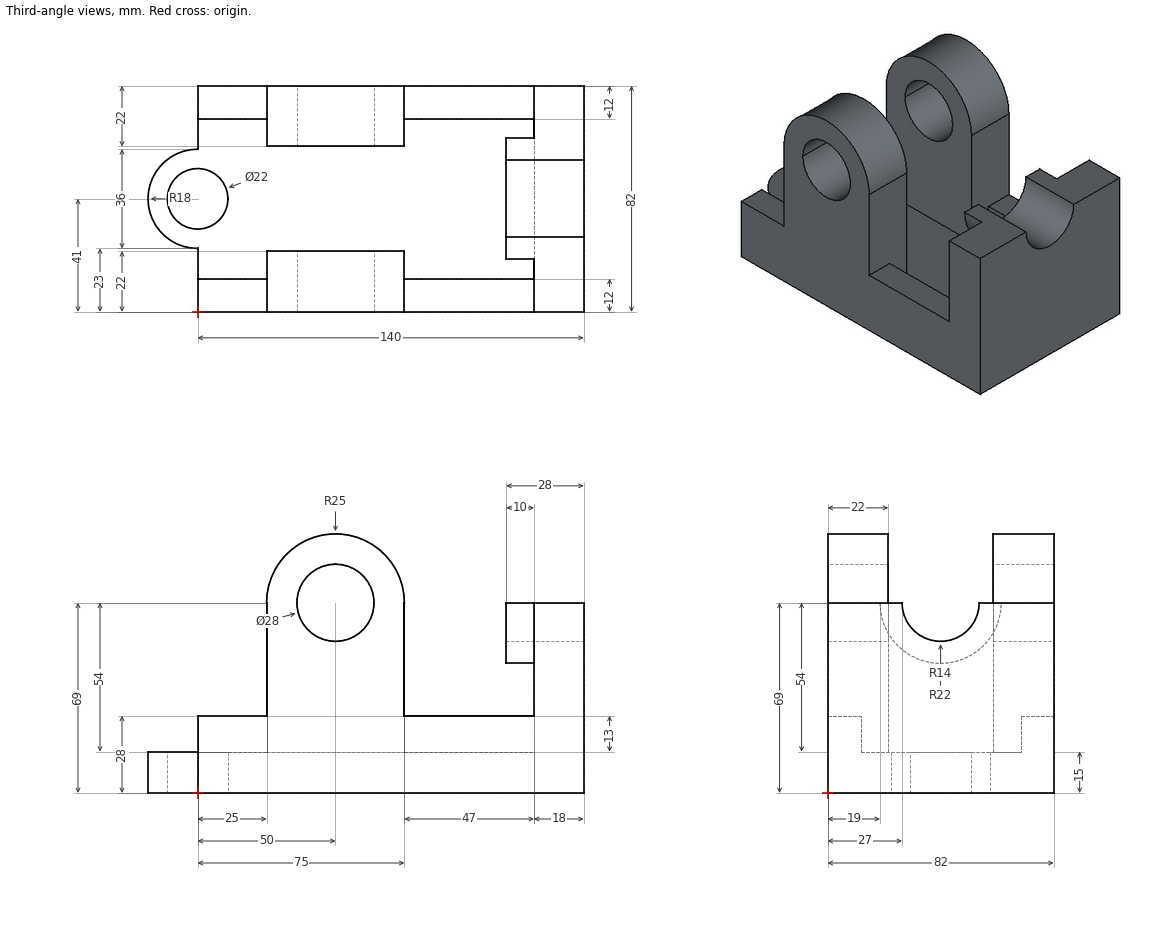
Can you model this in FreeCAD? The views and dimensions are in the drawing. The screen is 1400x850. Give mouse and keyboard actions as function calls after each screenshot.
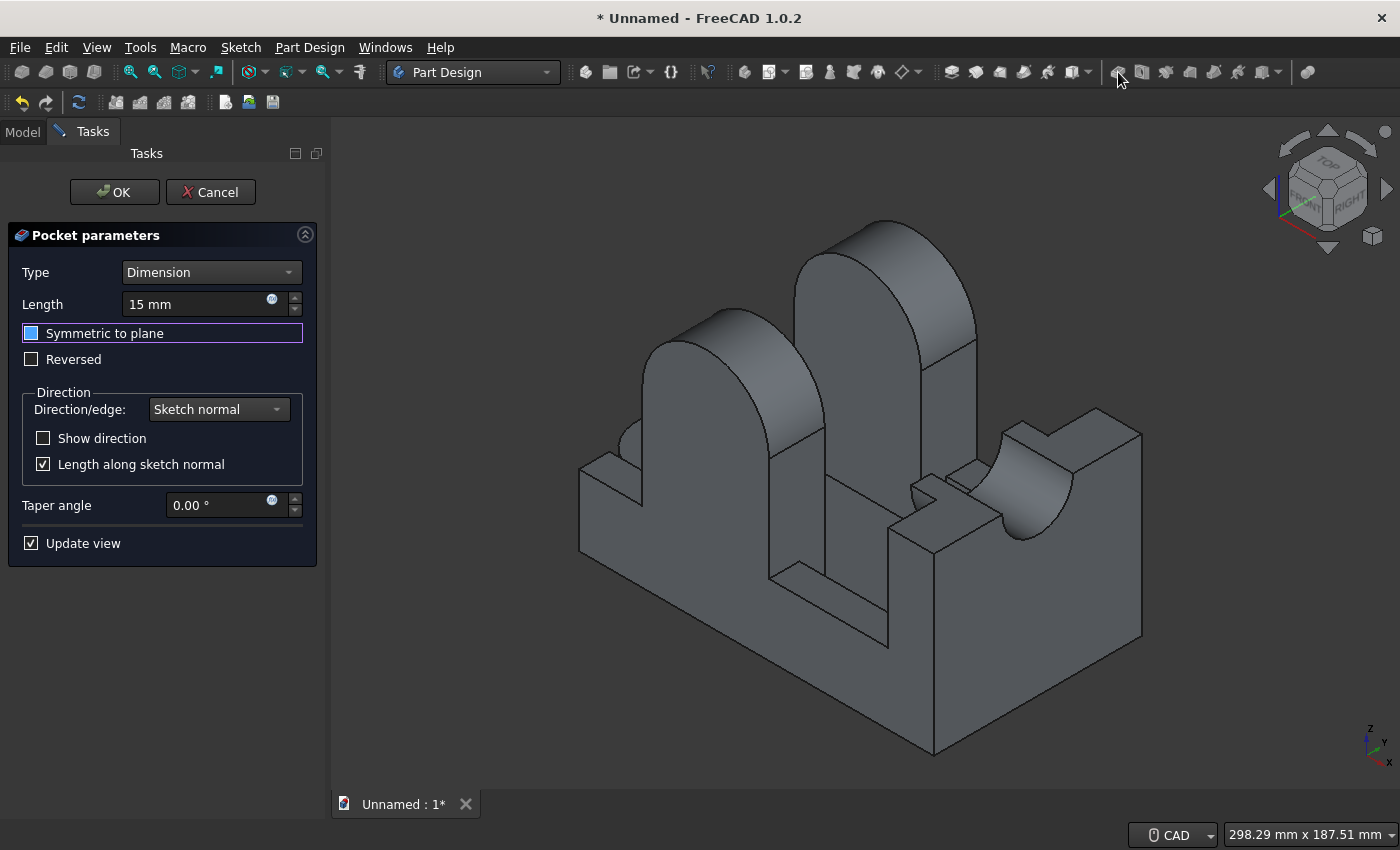
click(115, 192)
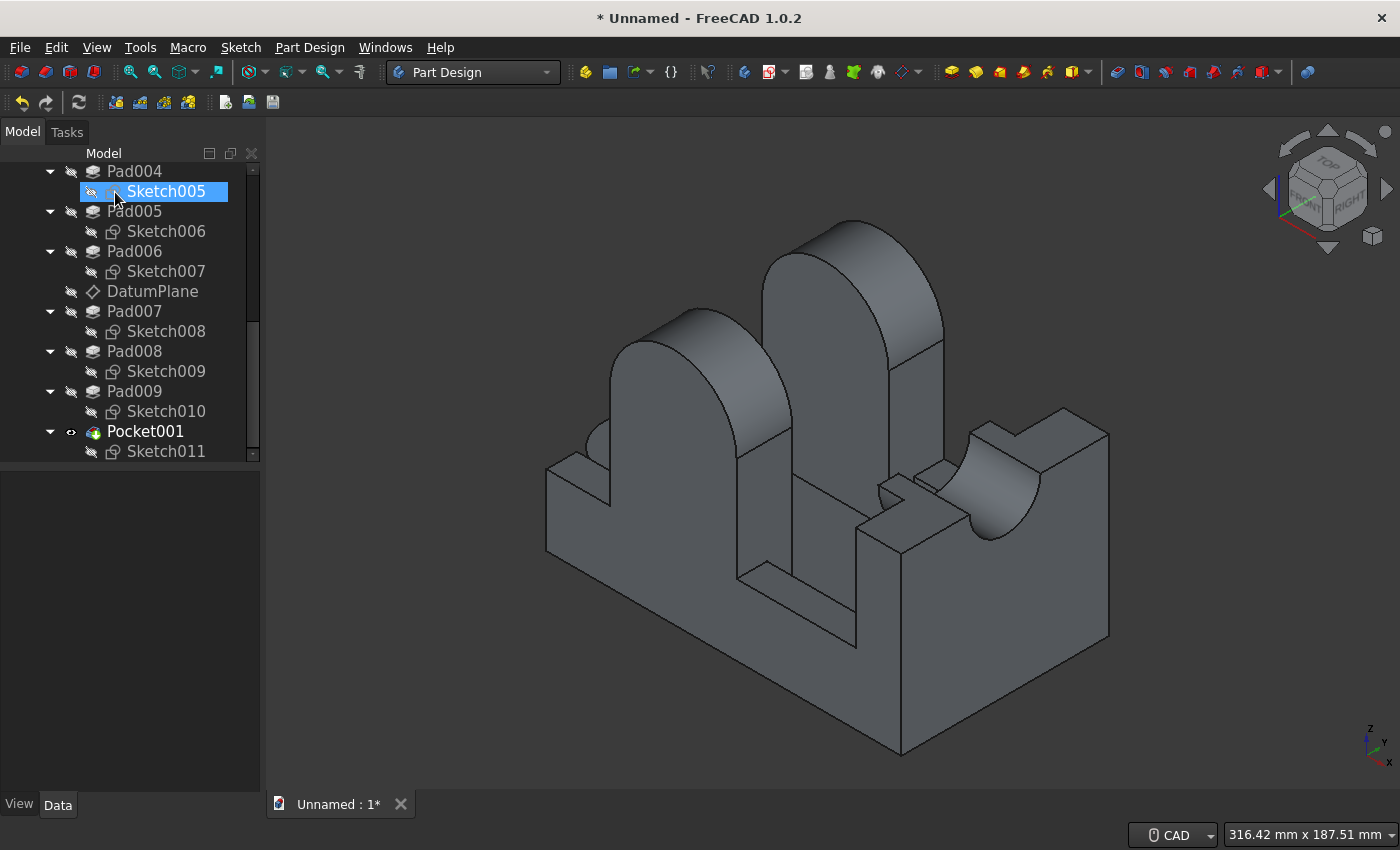
key(4)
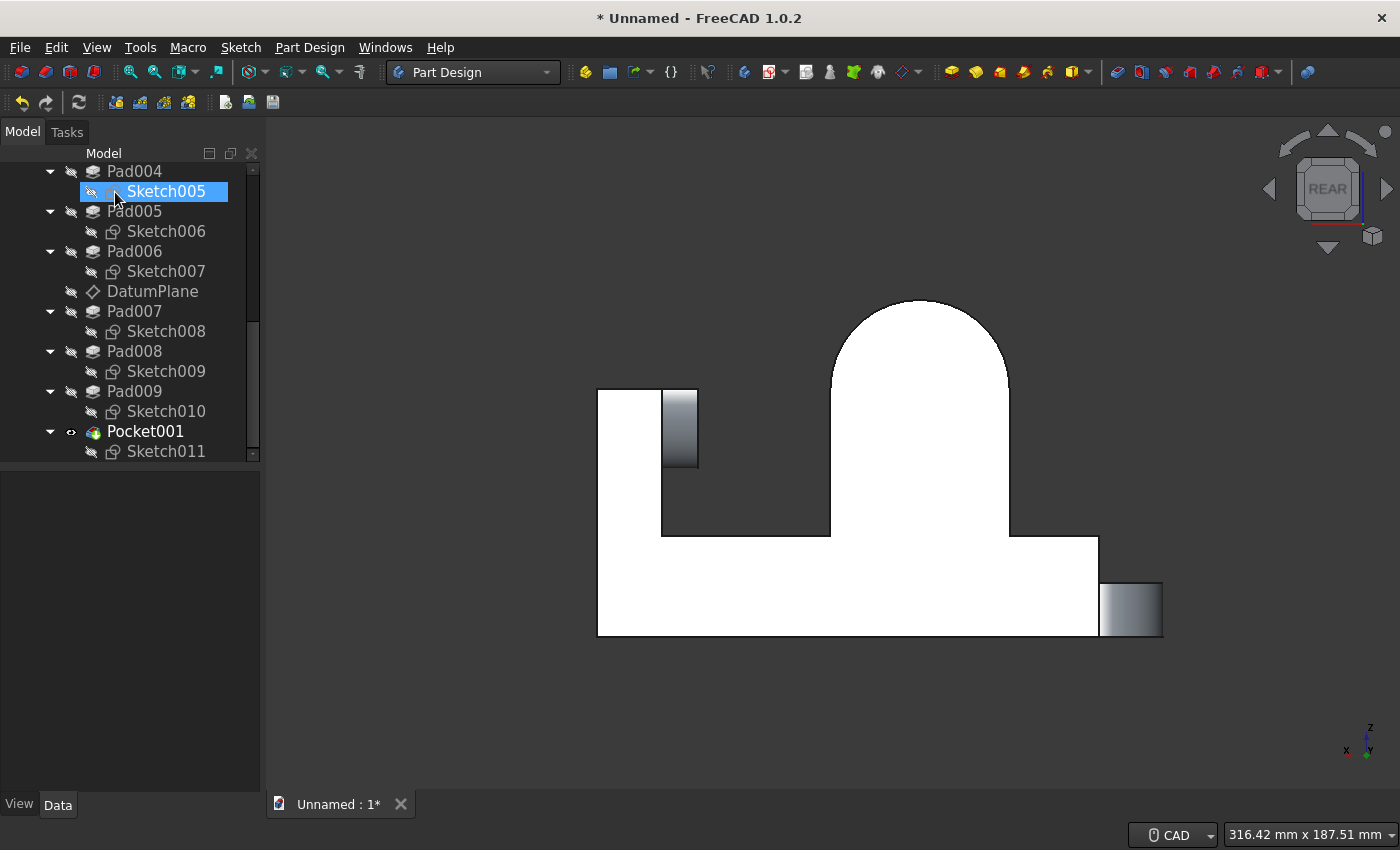
click(920, 419)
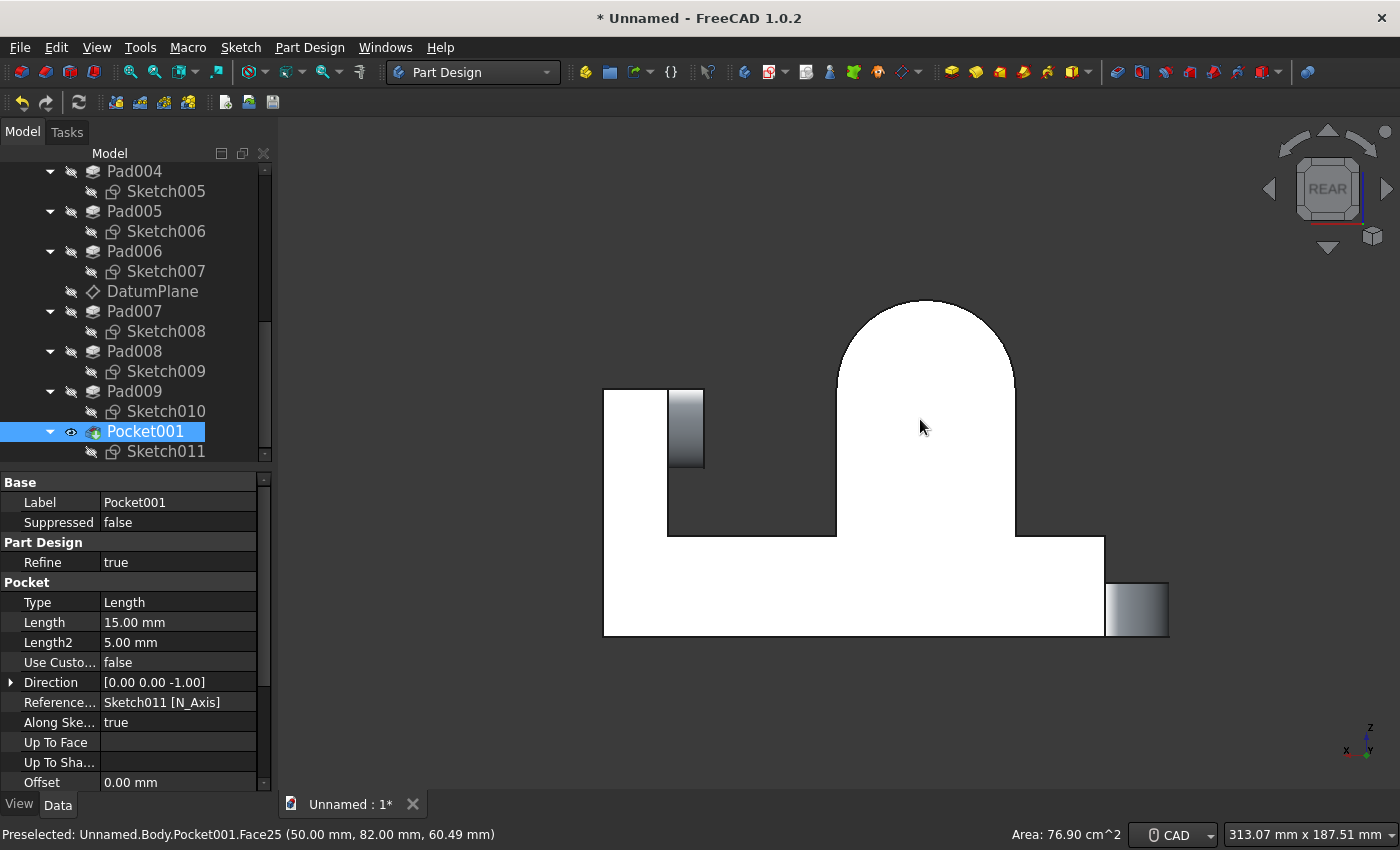
click(770, 72)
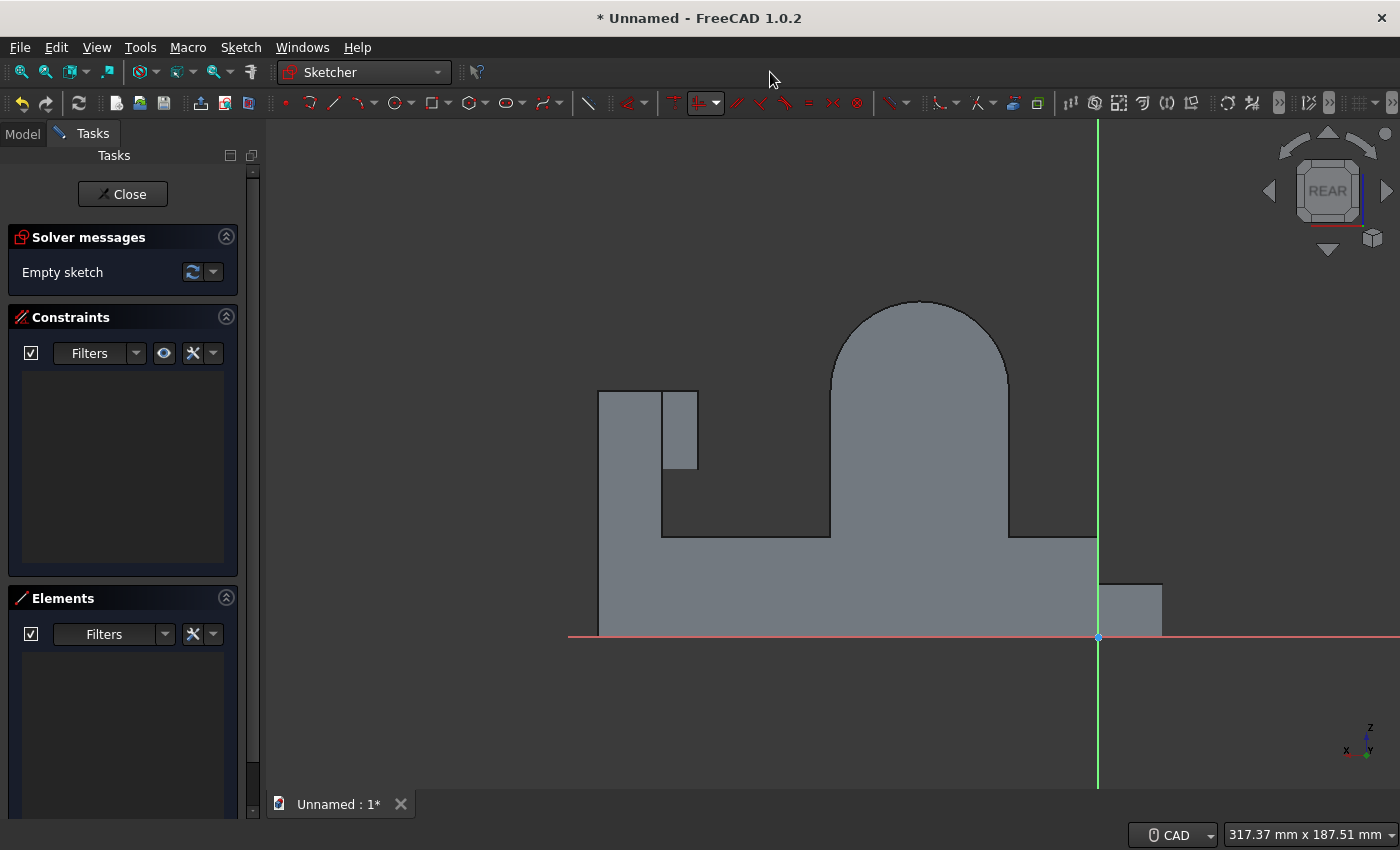
scroll(971, 370, up, 7)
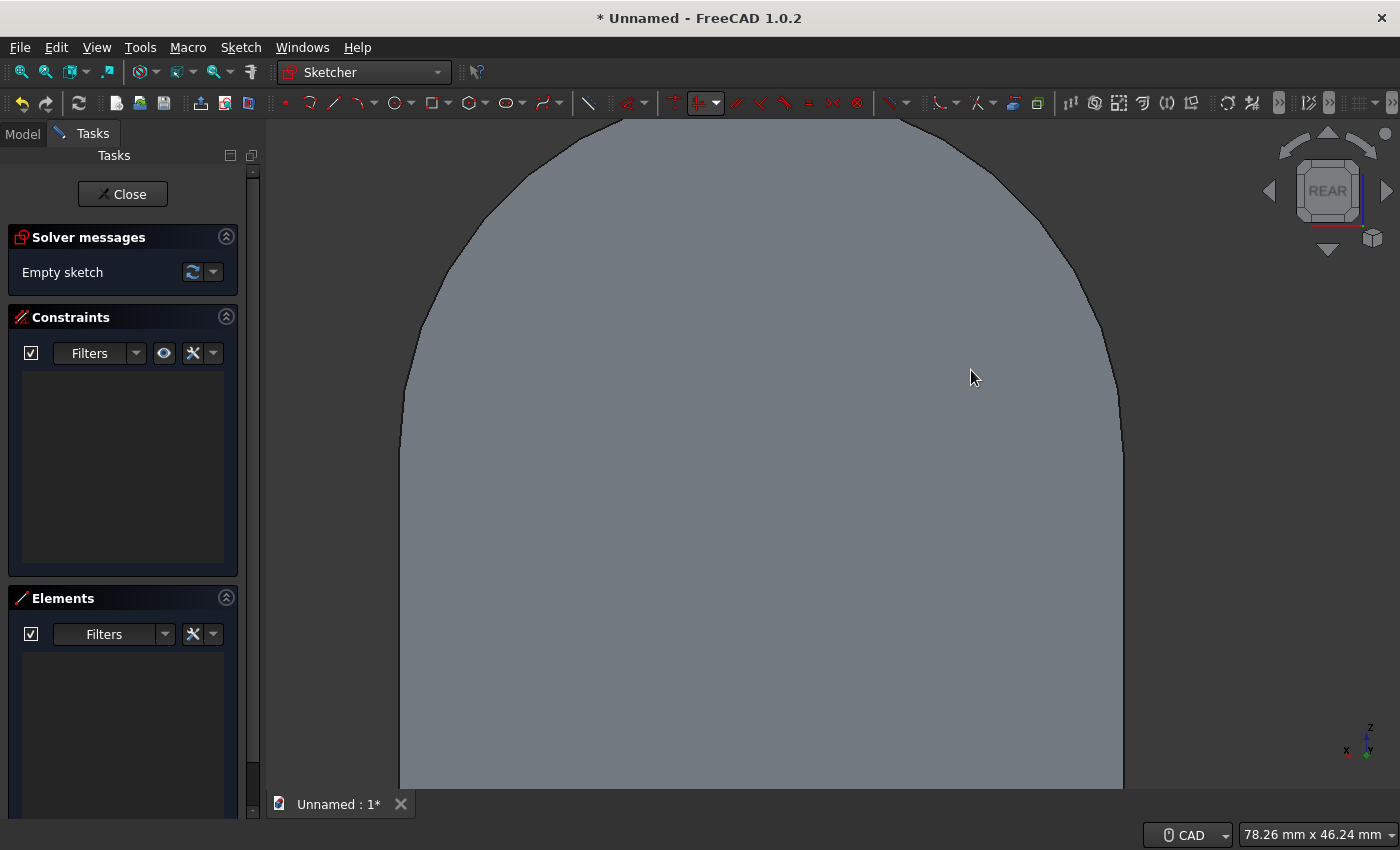
click(396, 104)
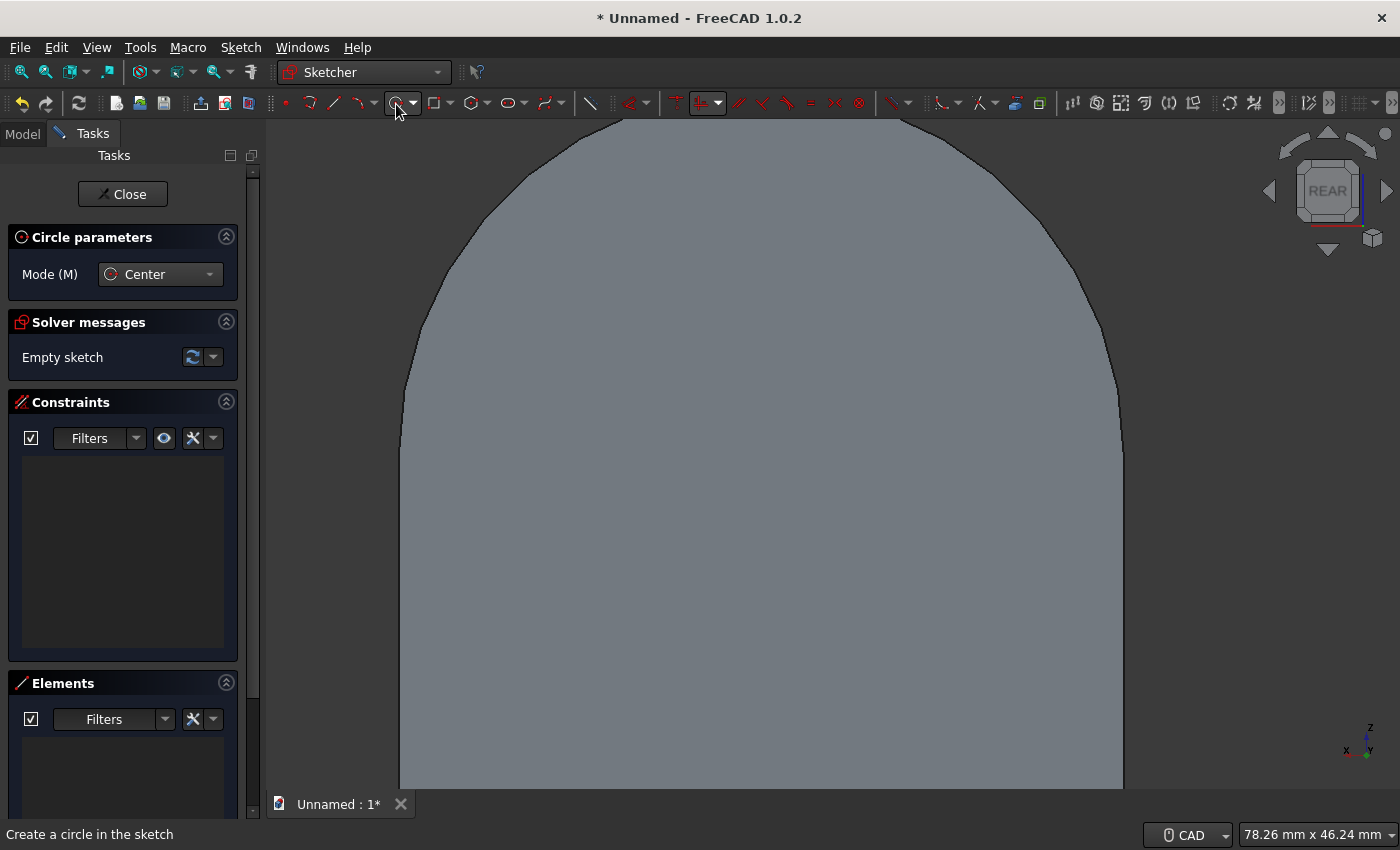
click(761, 453)
click(905, 309)
key(Escape)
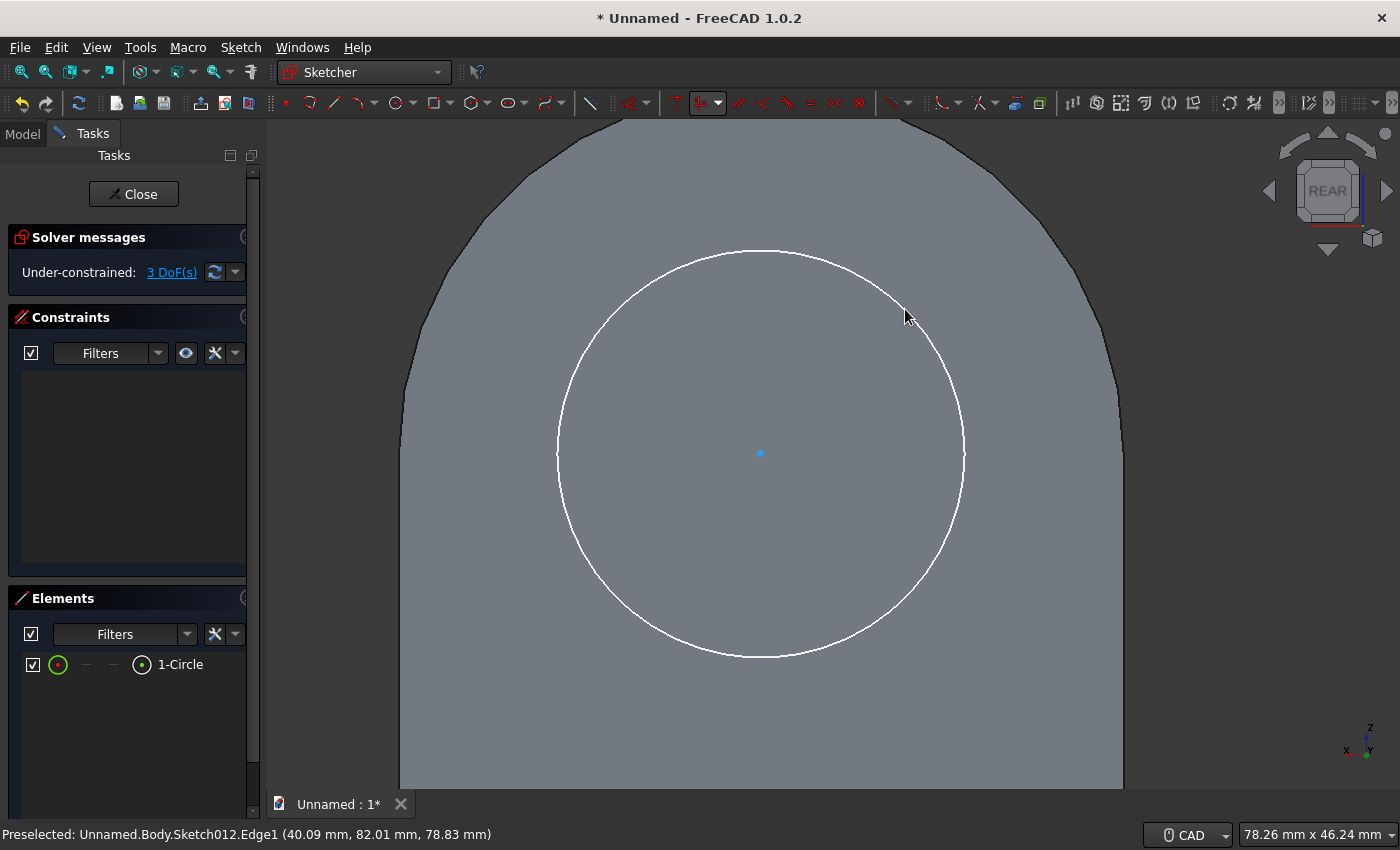
click(630, 104)